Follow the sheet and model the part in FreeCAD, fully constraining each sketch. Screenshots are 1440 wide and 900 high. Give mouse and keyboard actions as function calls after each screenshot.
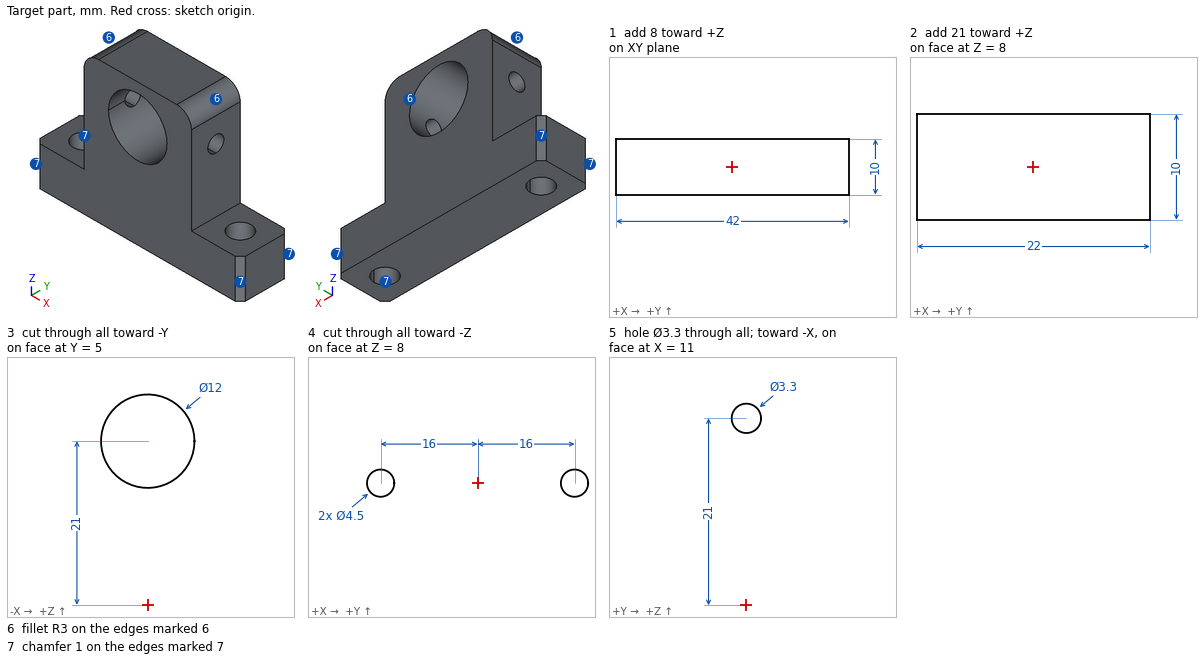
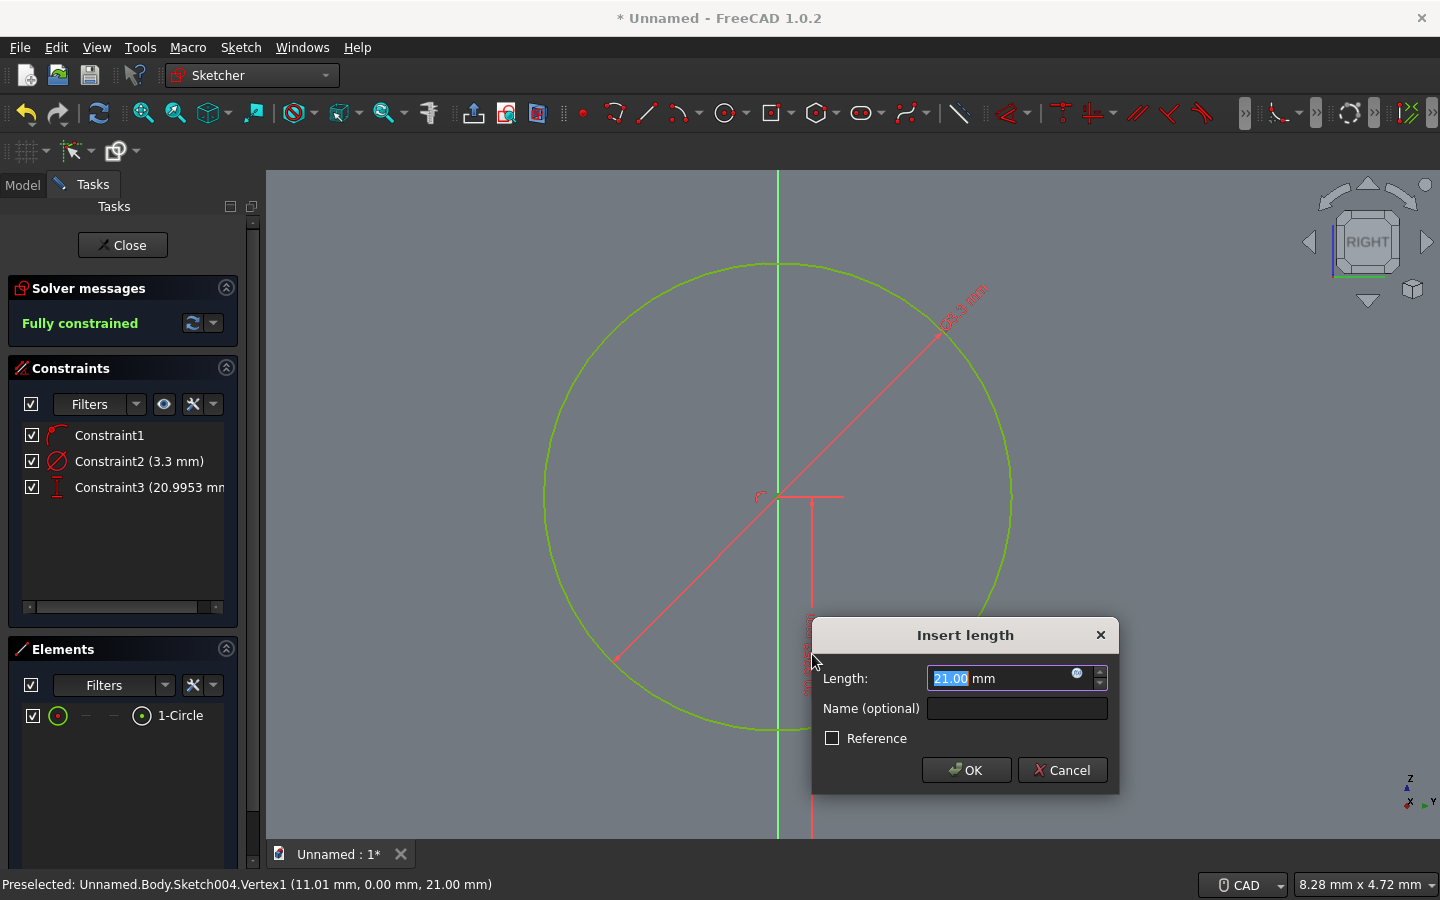
text(21)
key(Return)
key(Escape)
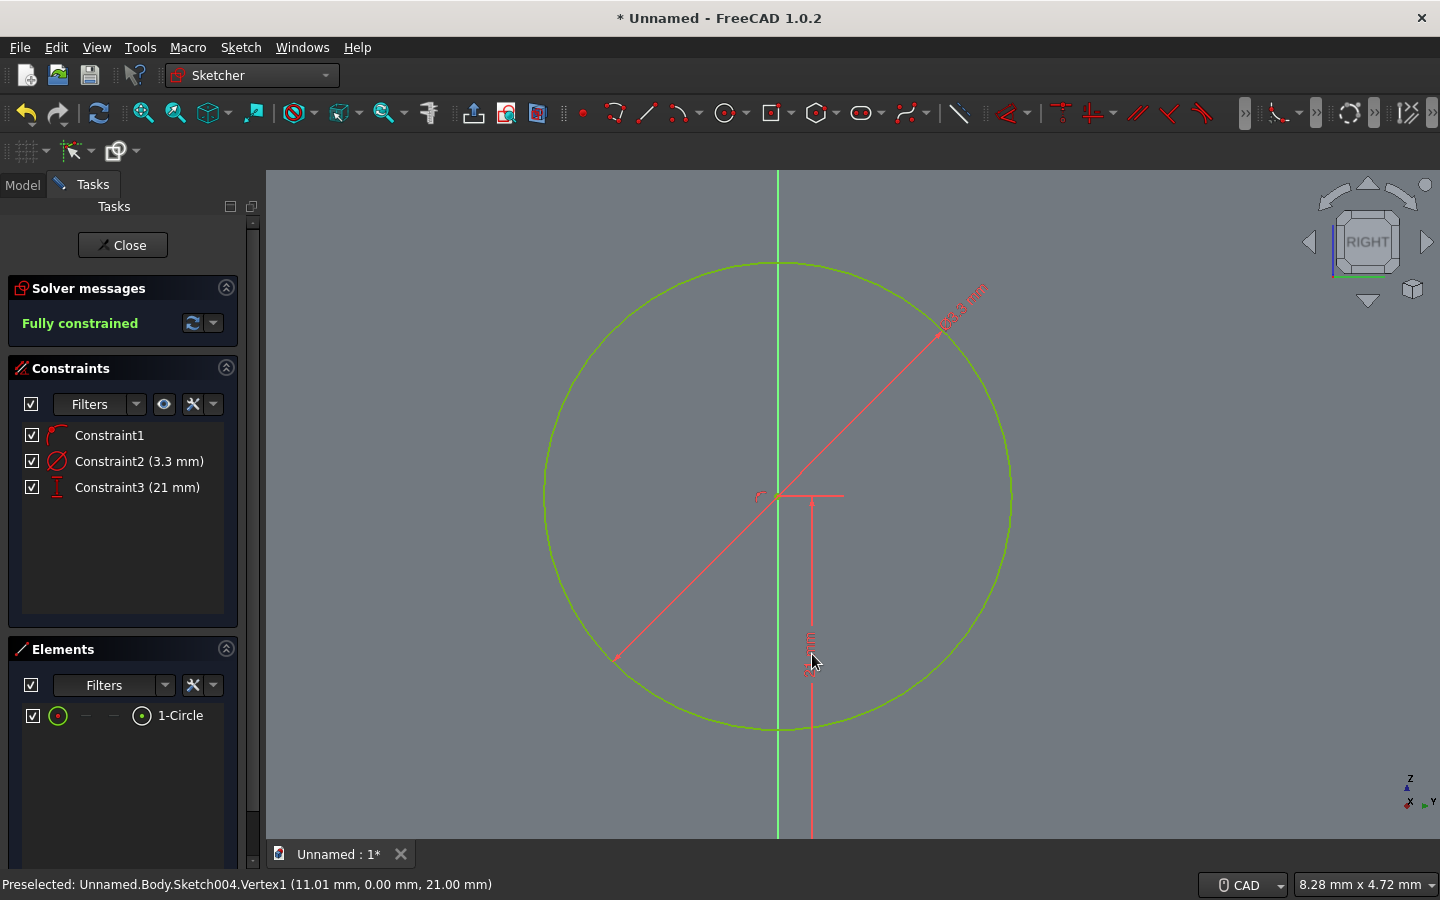
click(123, 245)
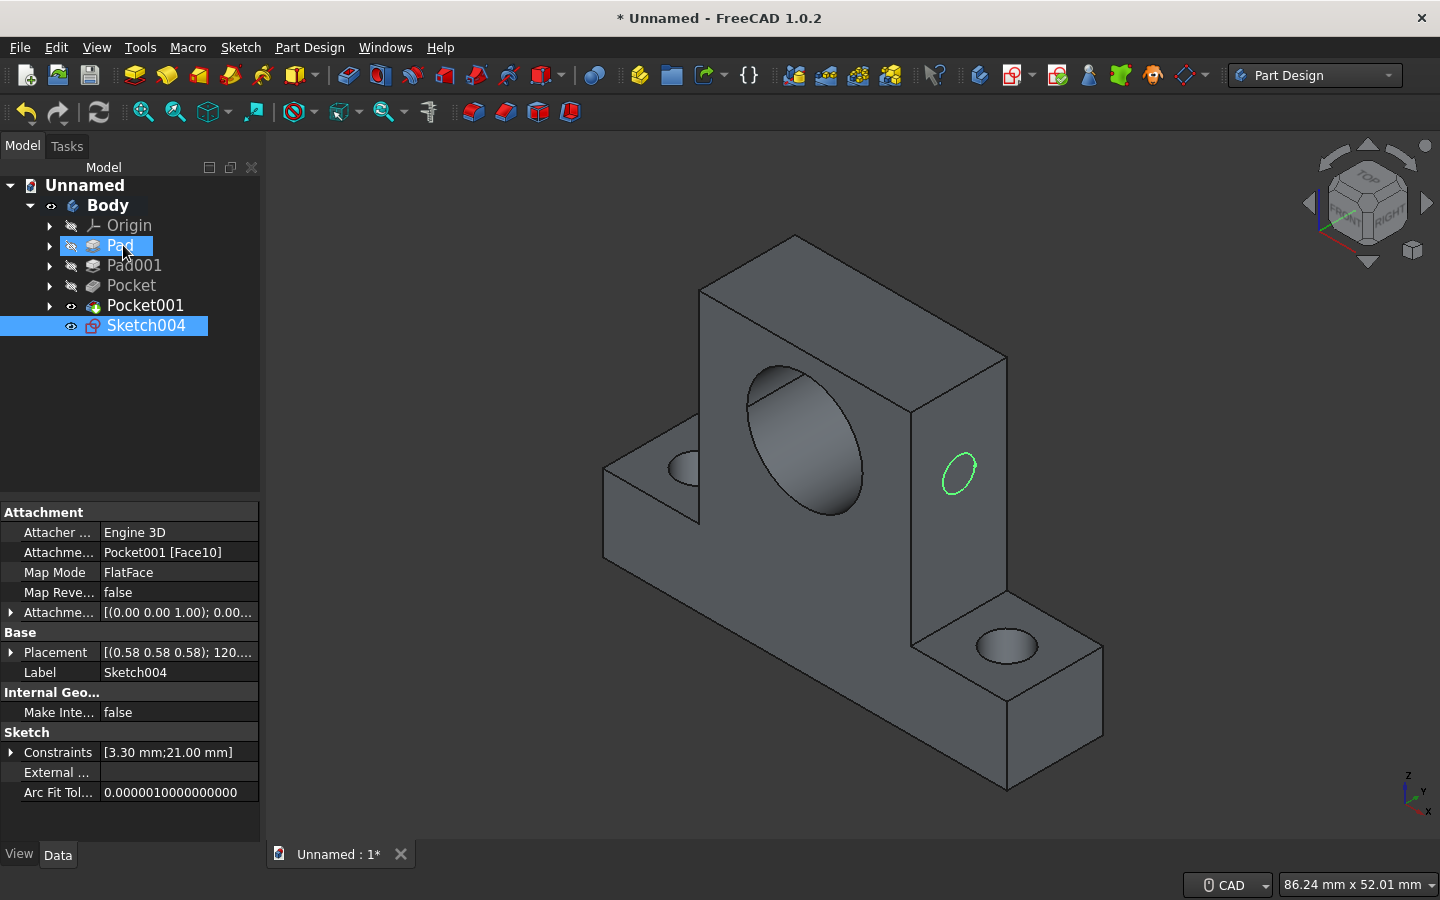
click(382, 76)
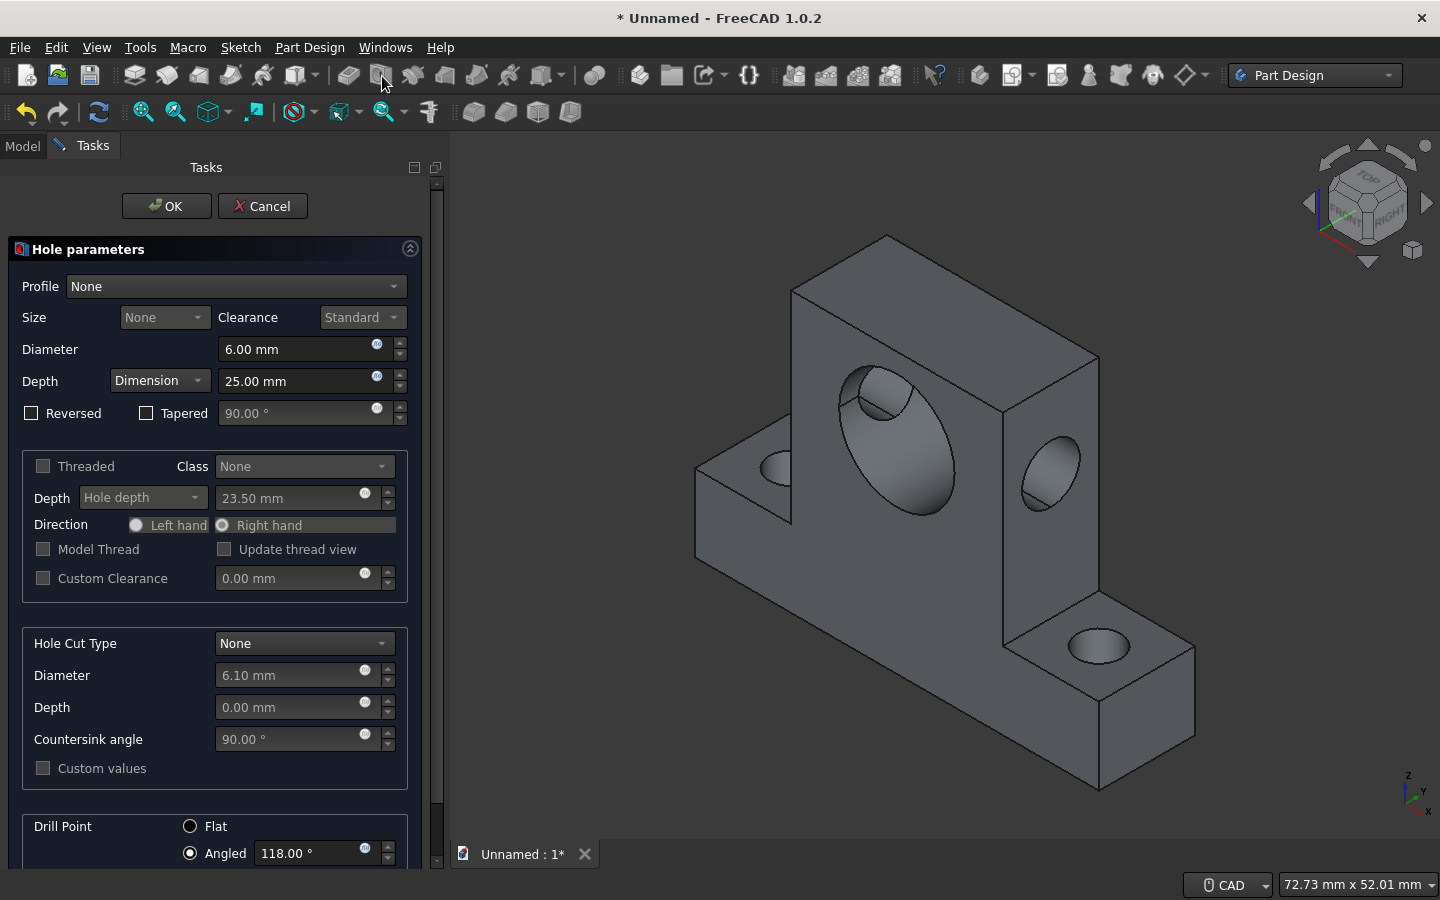
triple_click(305, 349)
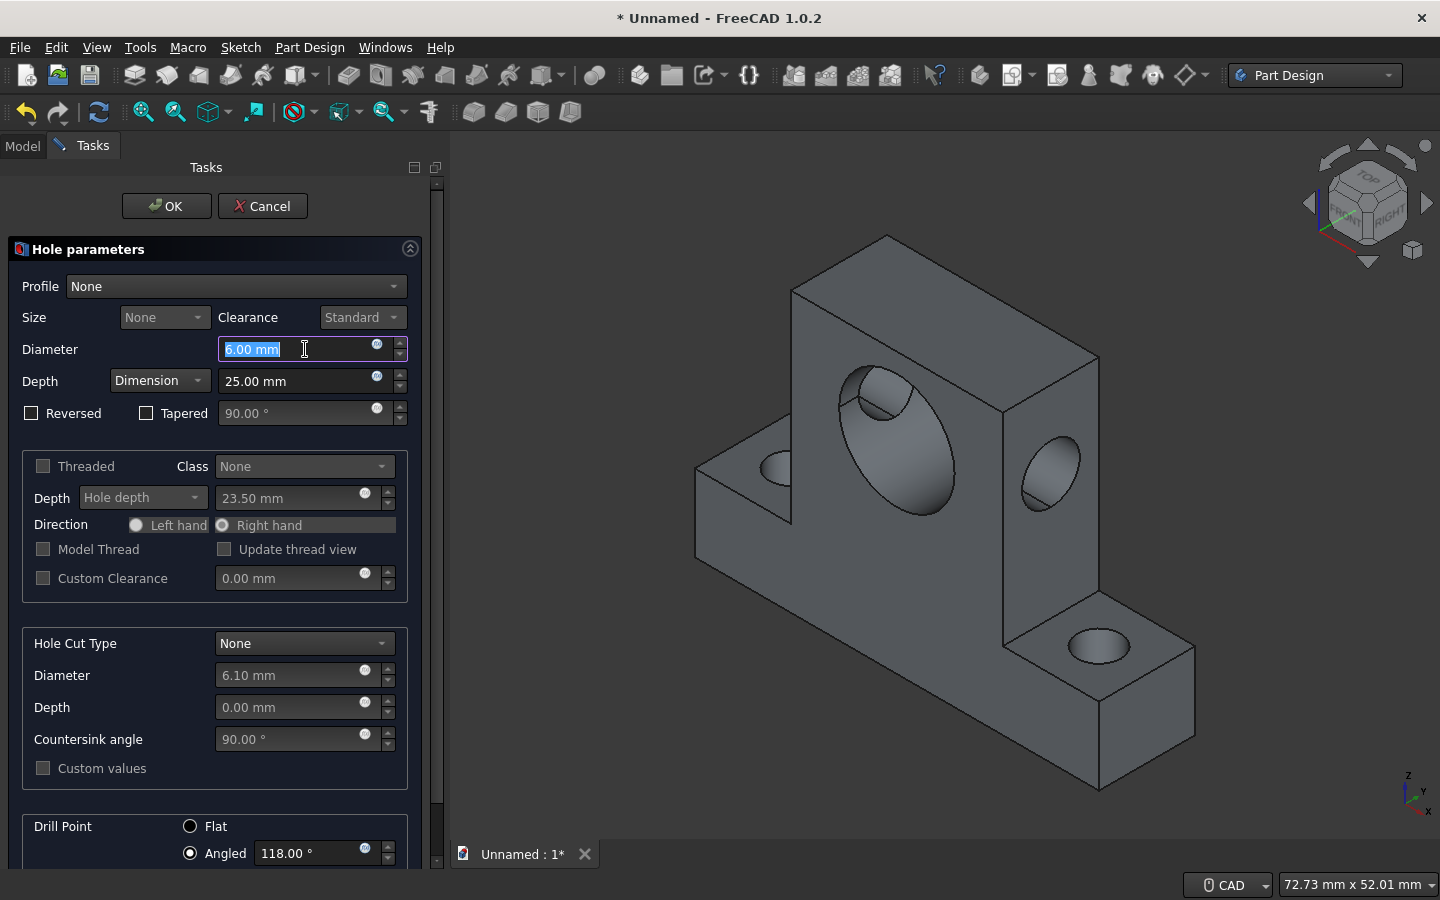
text(3.3)
key(Tab)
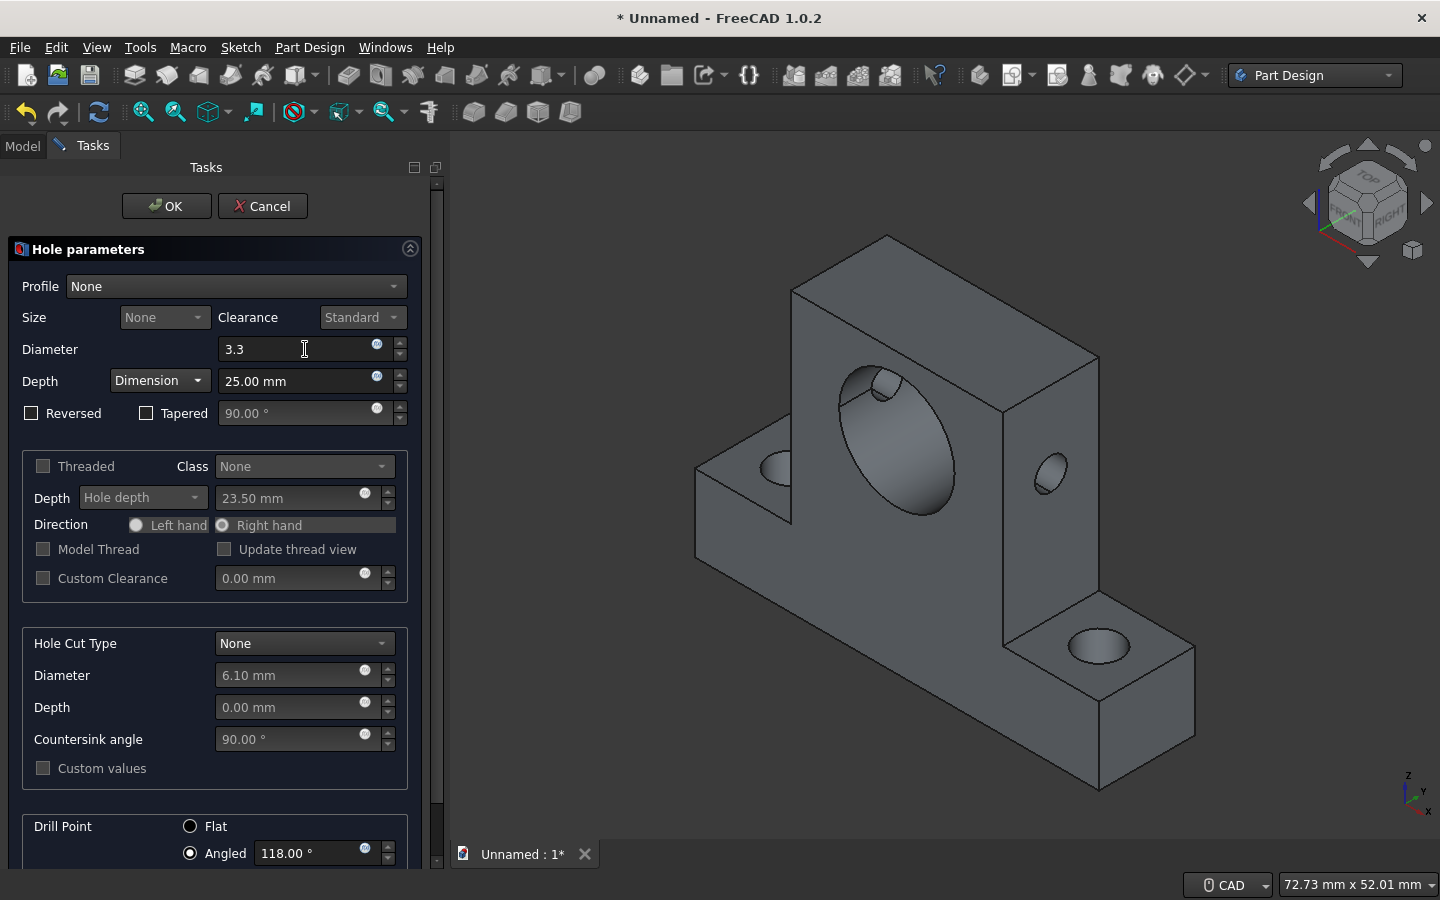
click(161, 380)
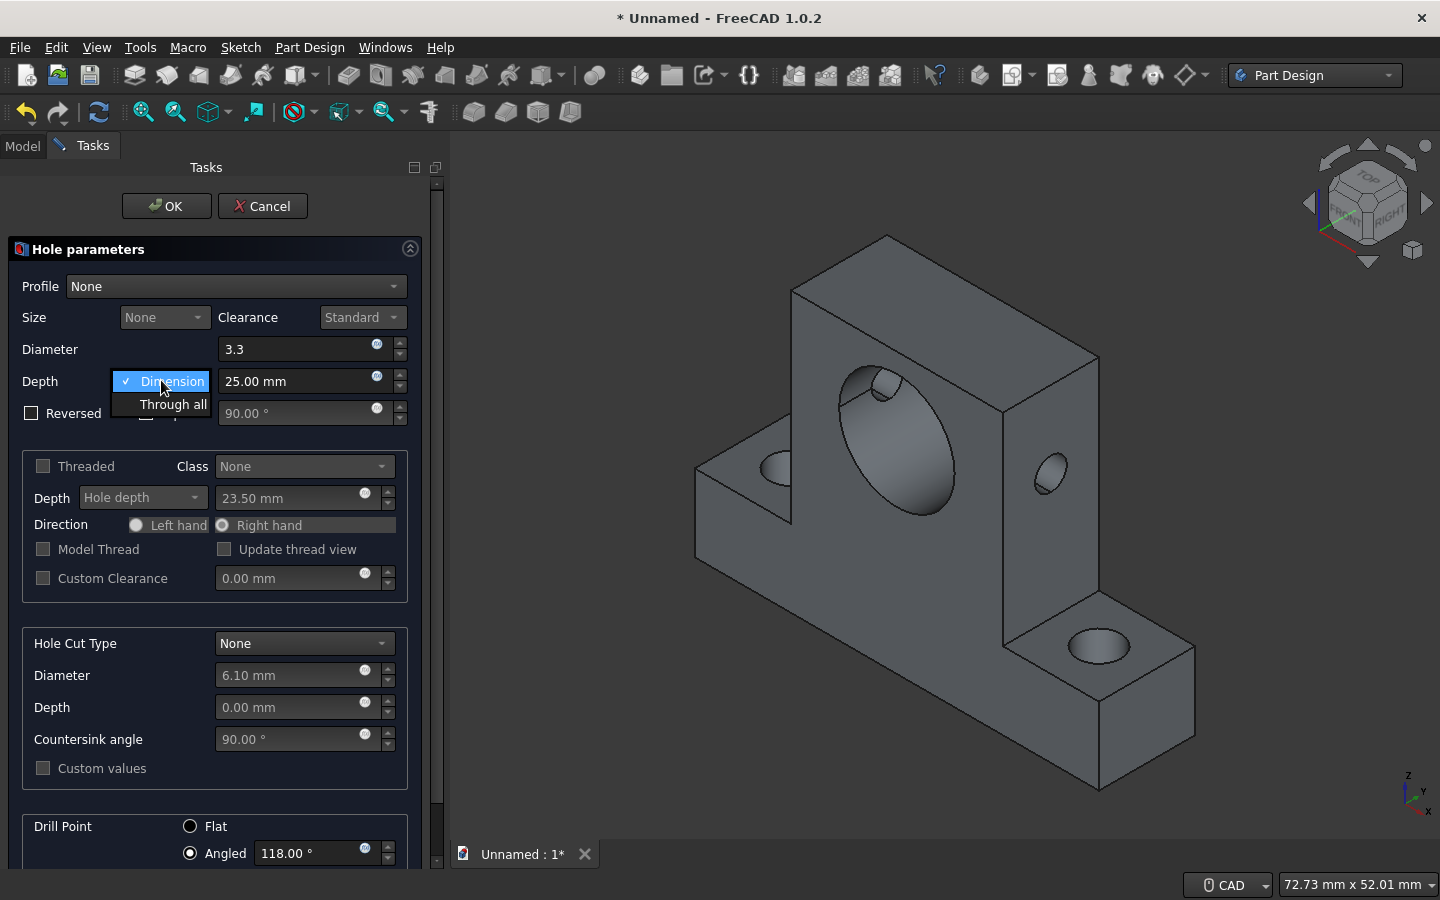
click(160, 404)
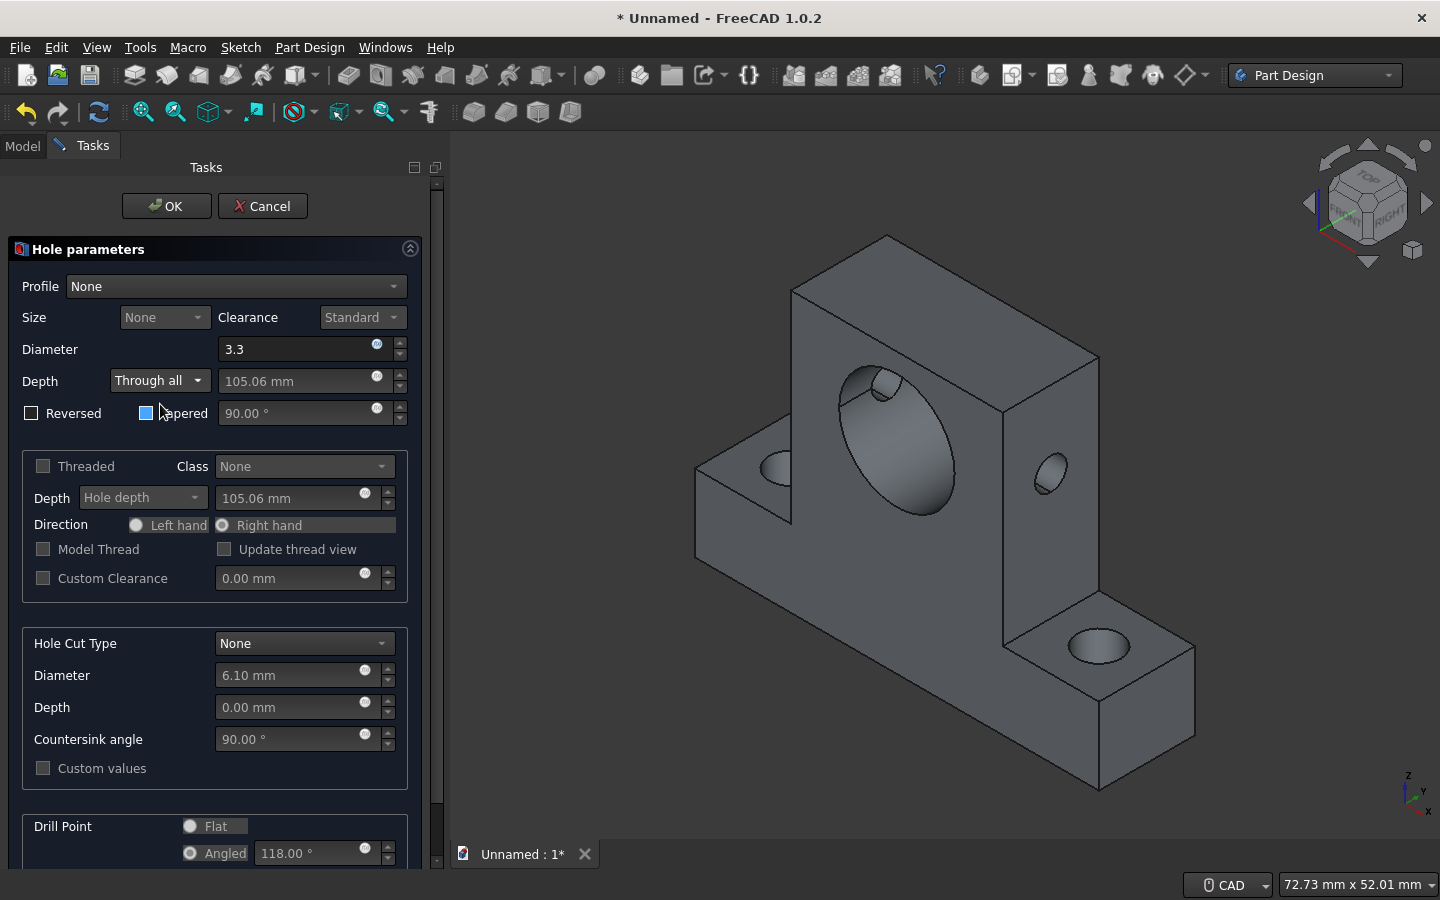
click(167, 206)